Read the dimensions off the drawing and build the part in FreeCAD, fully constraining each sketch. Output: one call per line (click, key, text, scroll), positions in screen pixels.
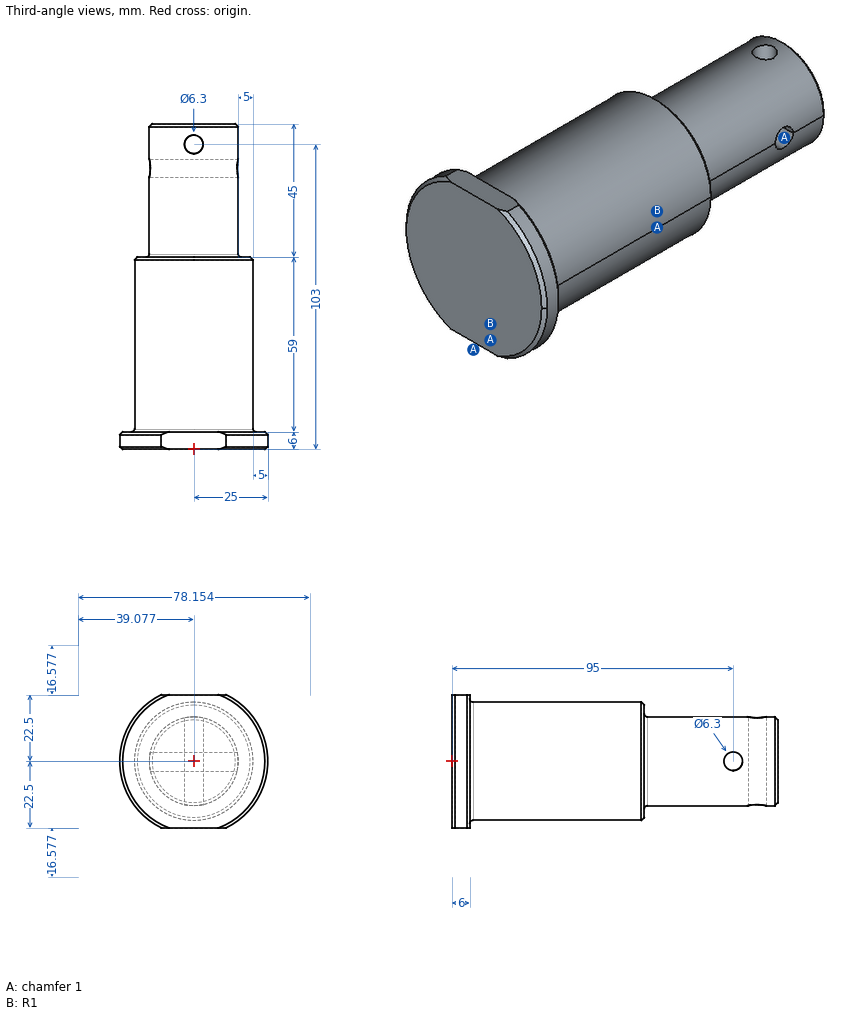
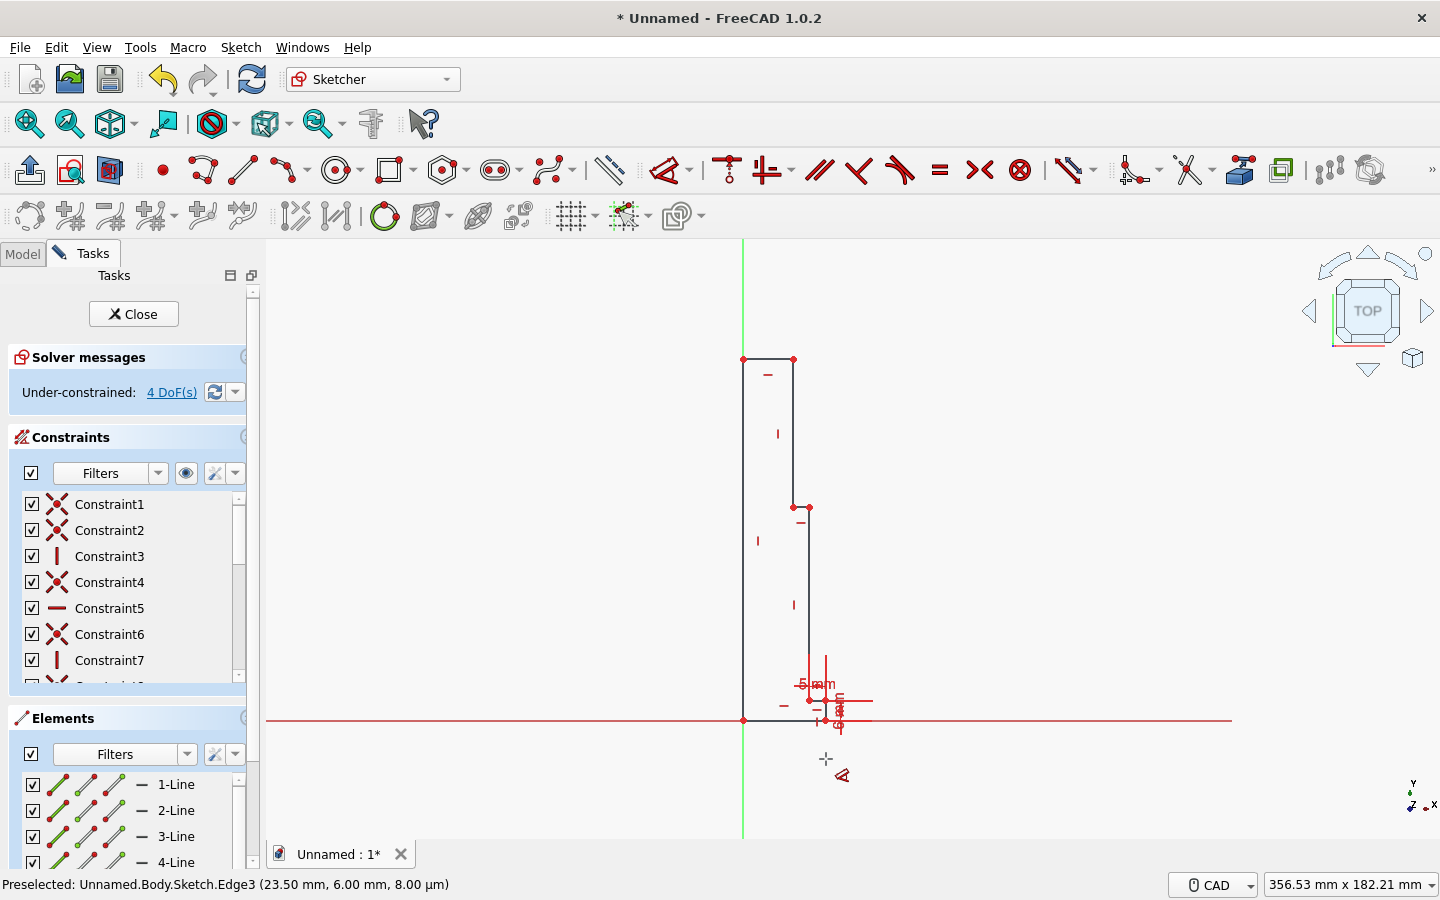
scroll(804, 507, up, 6)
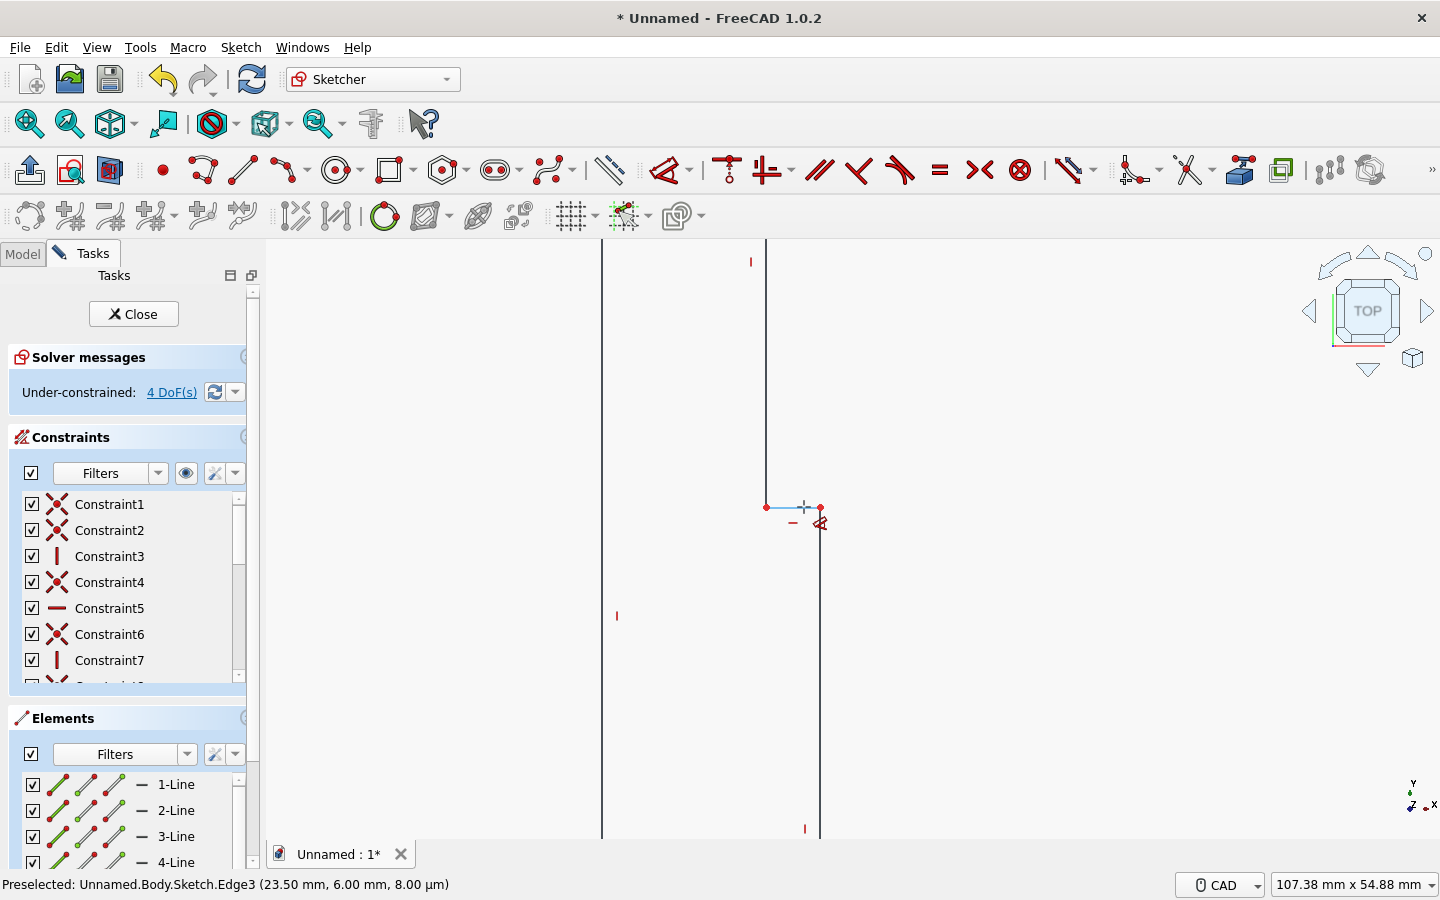
click(804, 508)
click(793, 474)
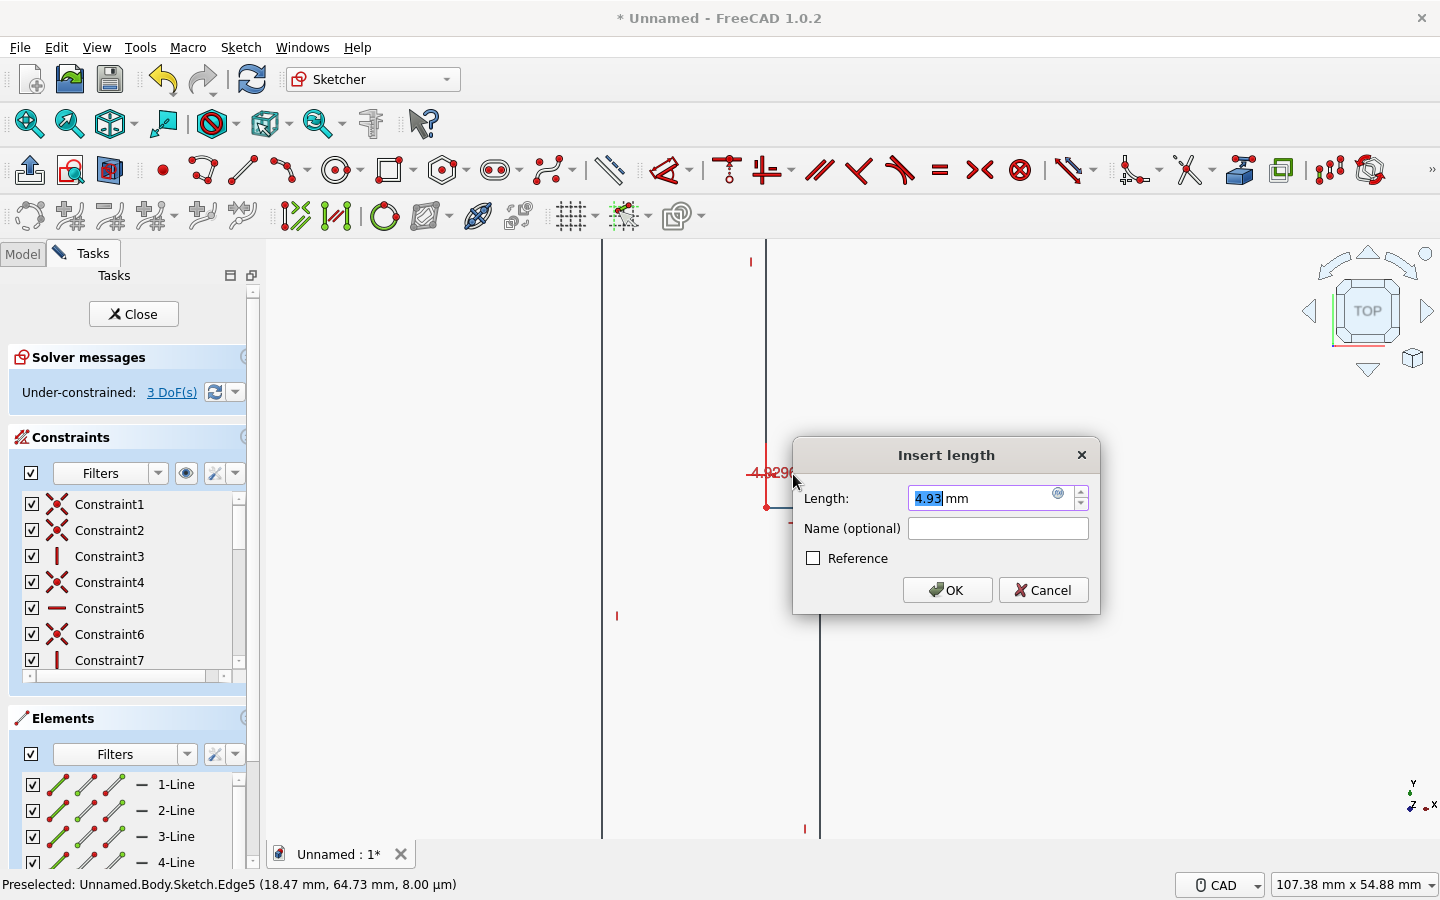
text(5)
key(Return)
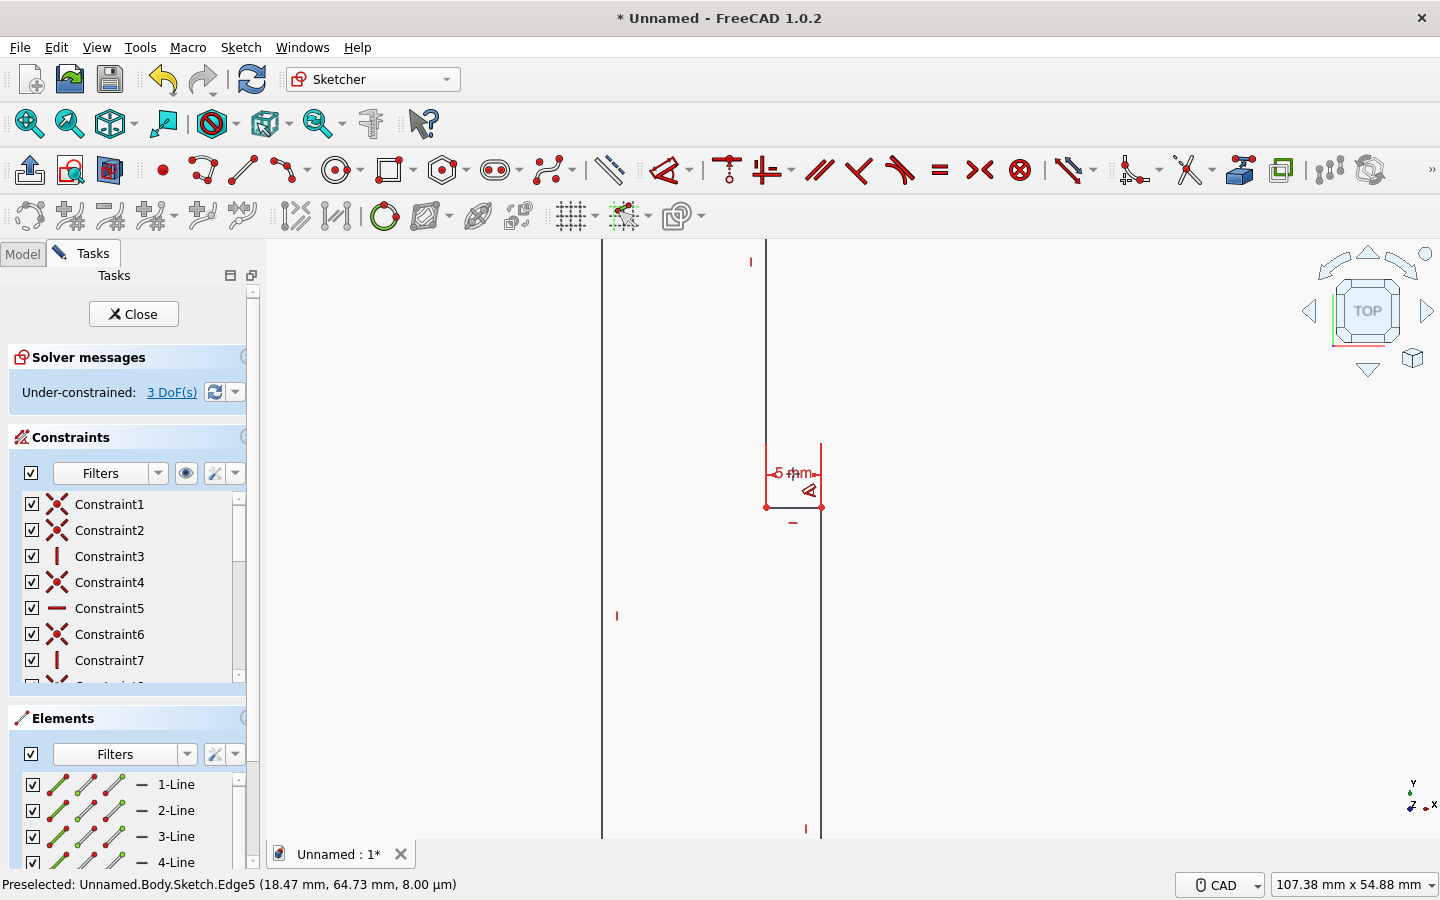
scroll(804, 507, down, 6)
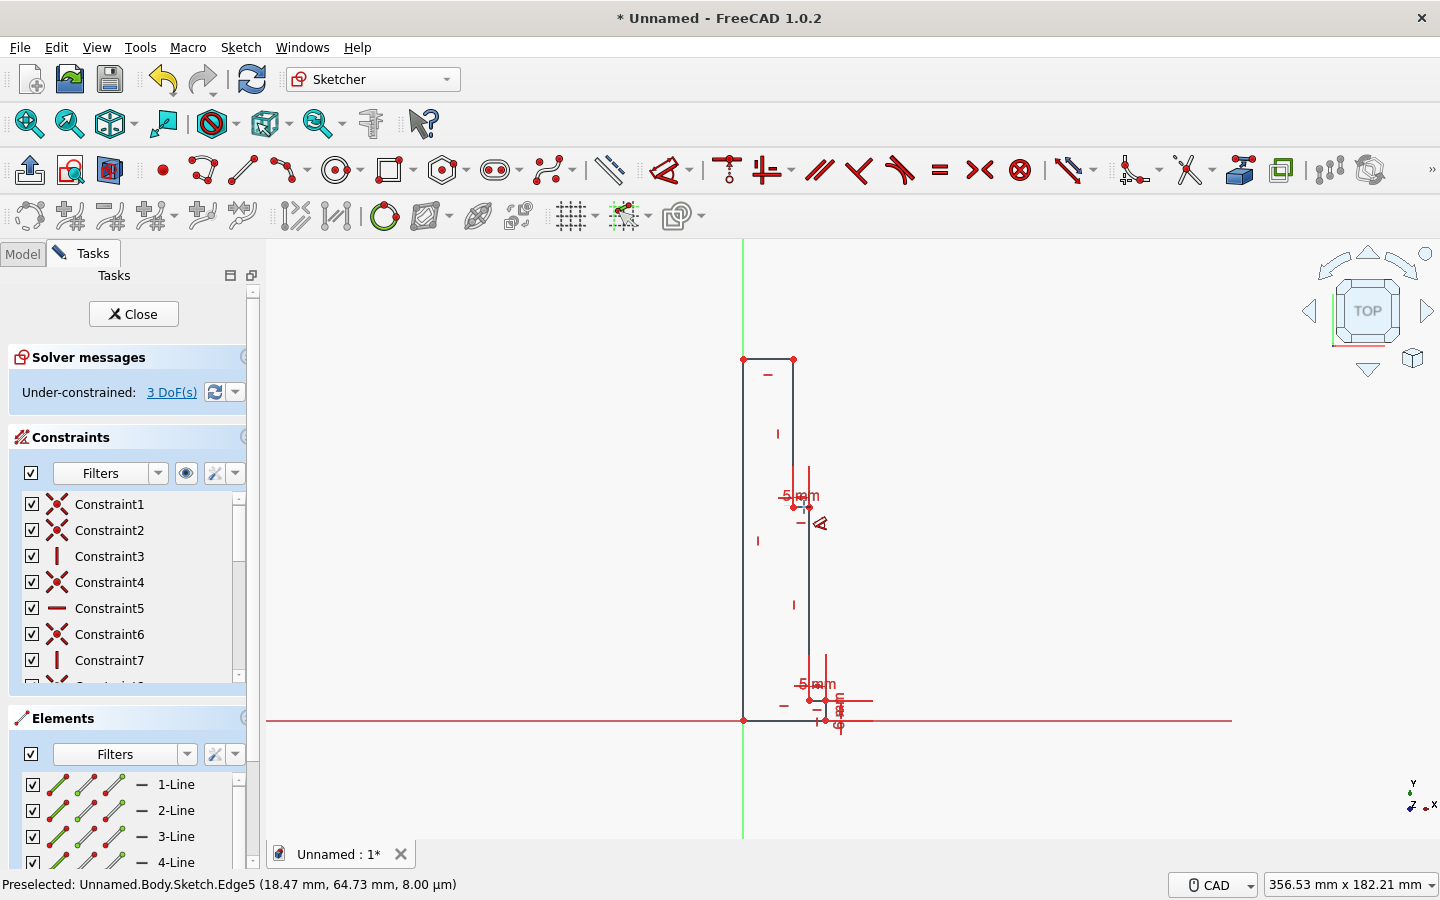
click(768, 721)
click(785, 755)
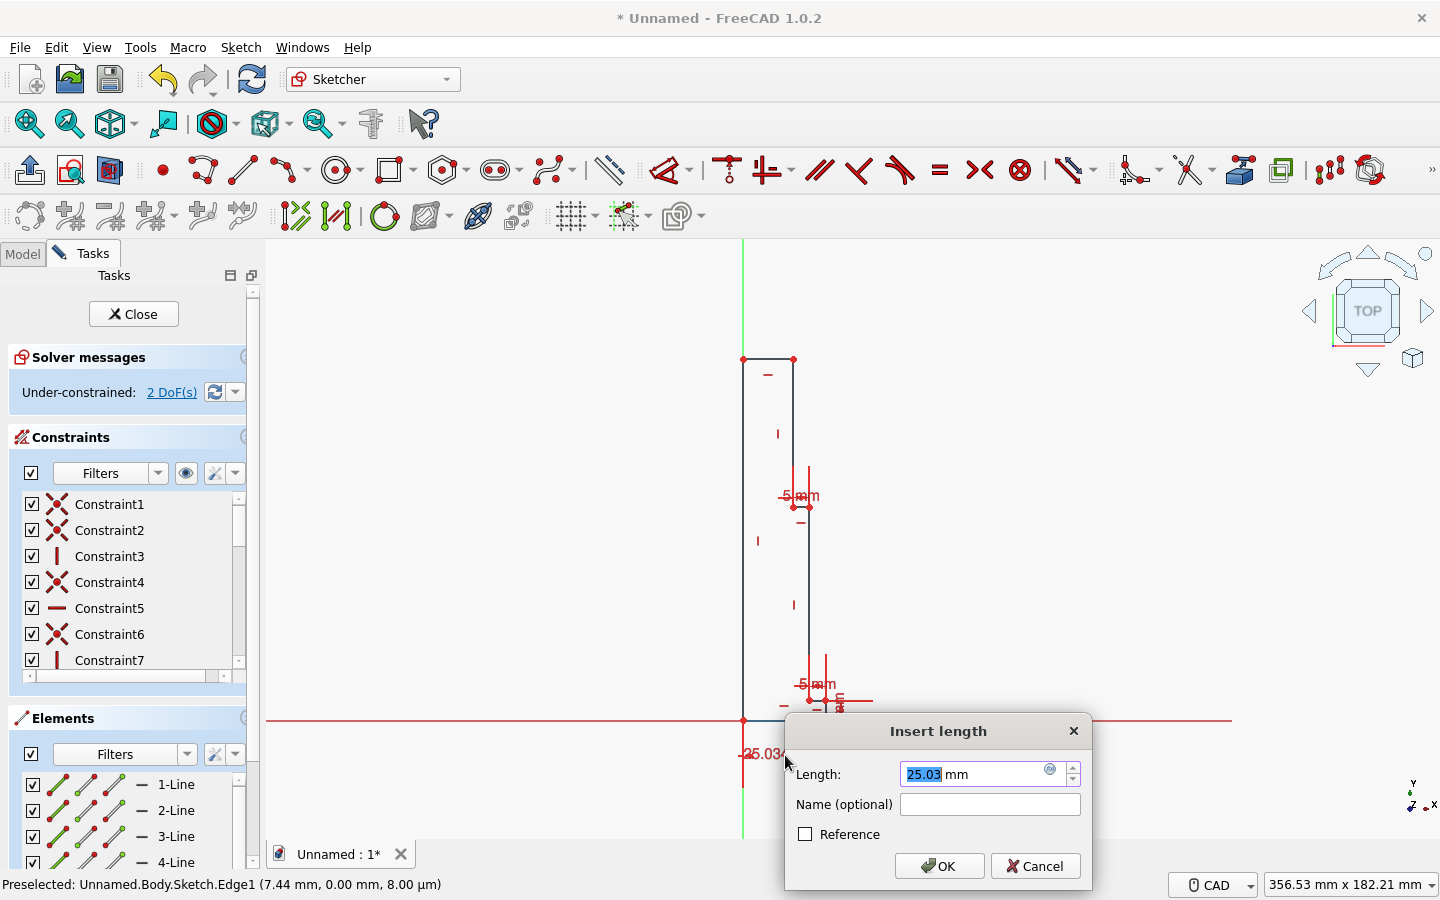
text(25)
key(Return)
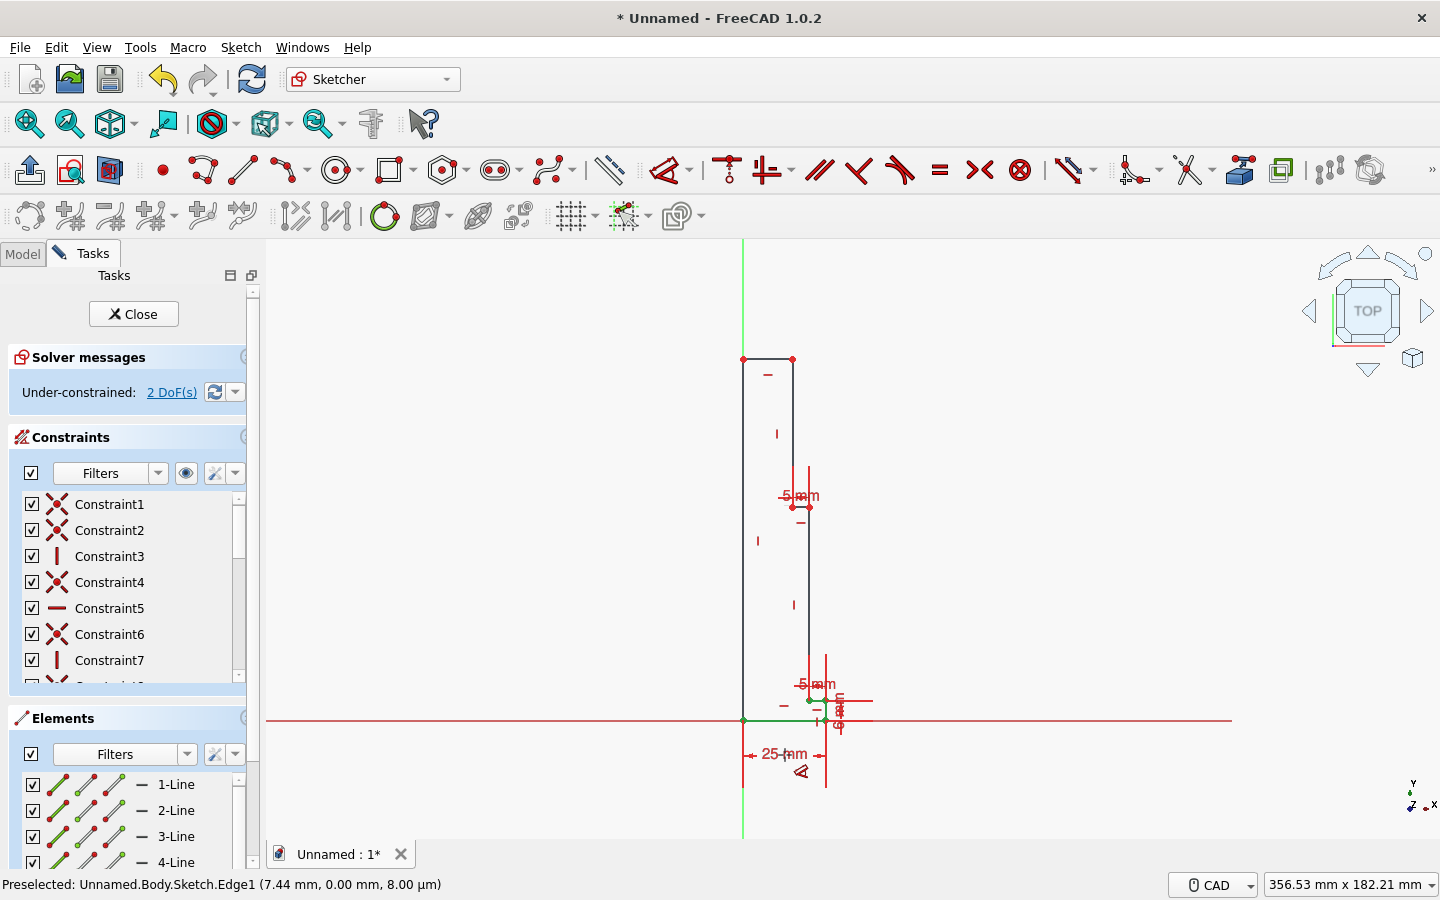
click(809, 643)
click(843, 604)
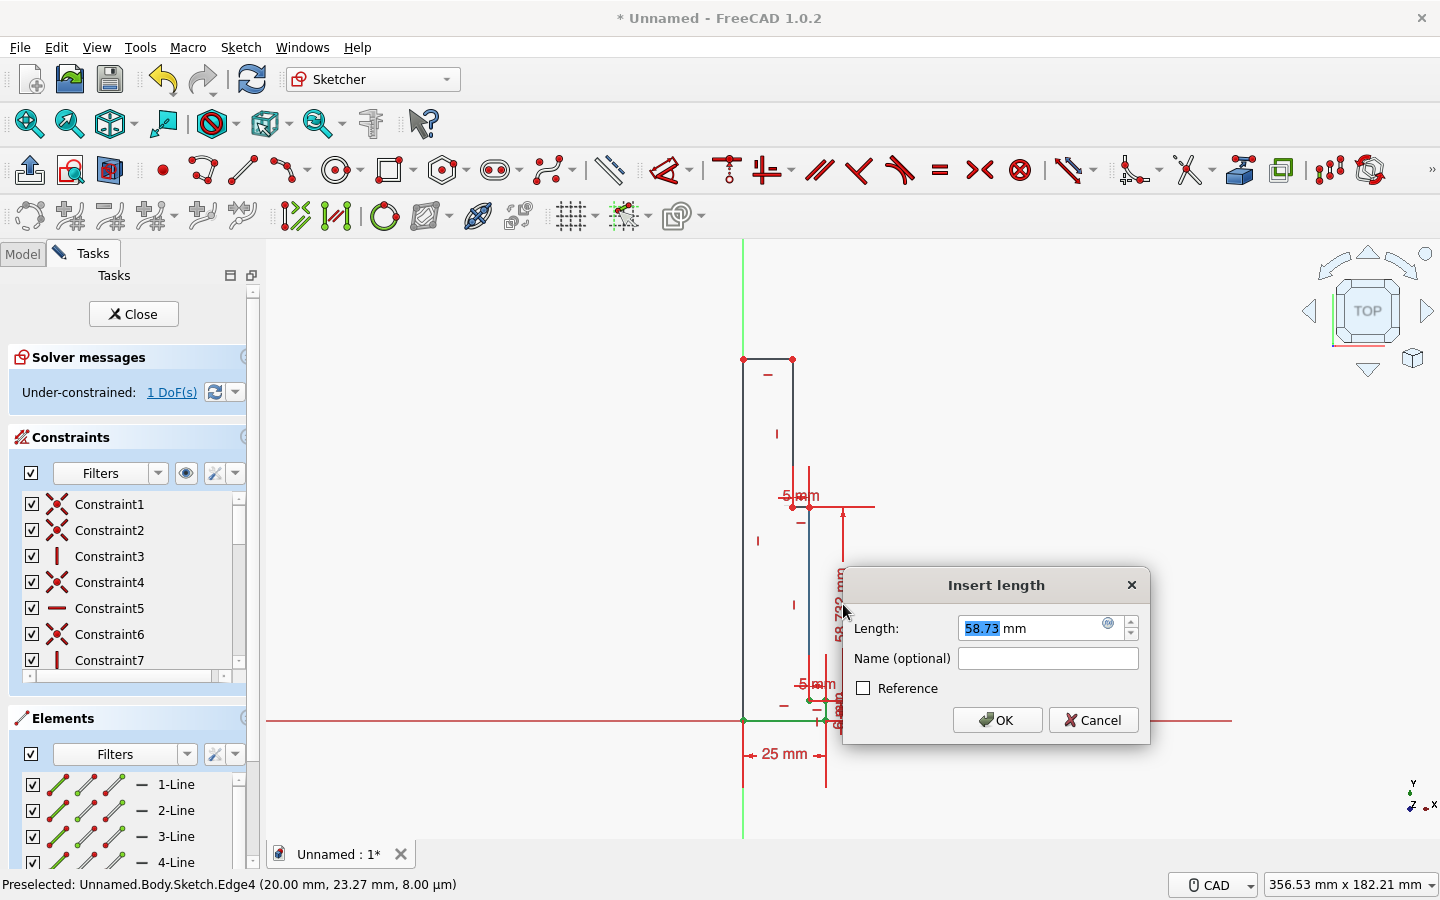
text(59)
key(Return)